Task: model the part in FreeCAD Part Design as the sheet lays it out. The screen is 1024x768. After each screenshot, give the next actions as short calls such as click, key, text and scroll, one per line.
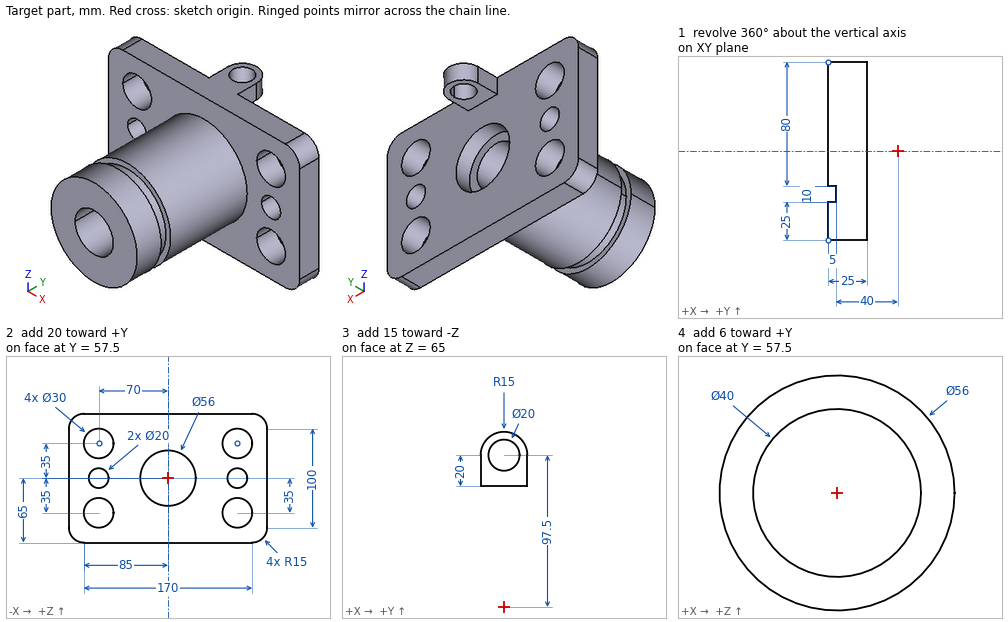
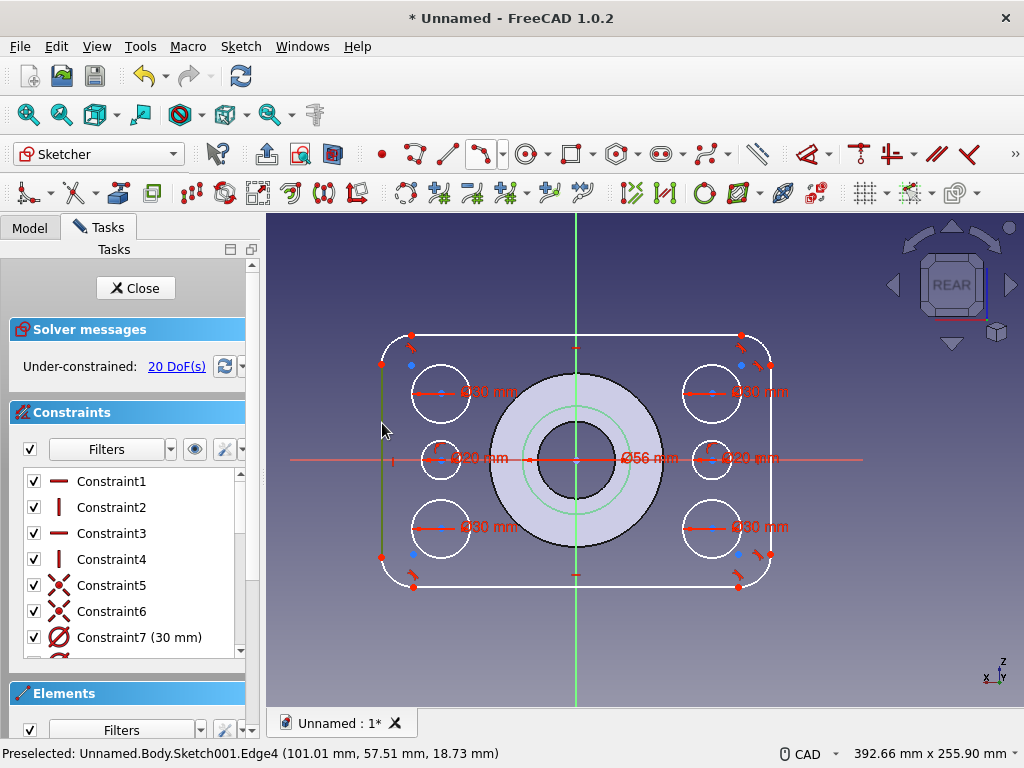
click(398, 339)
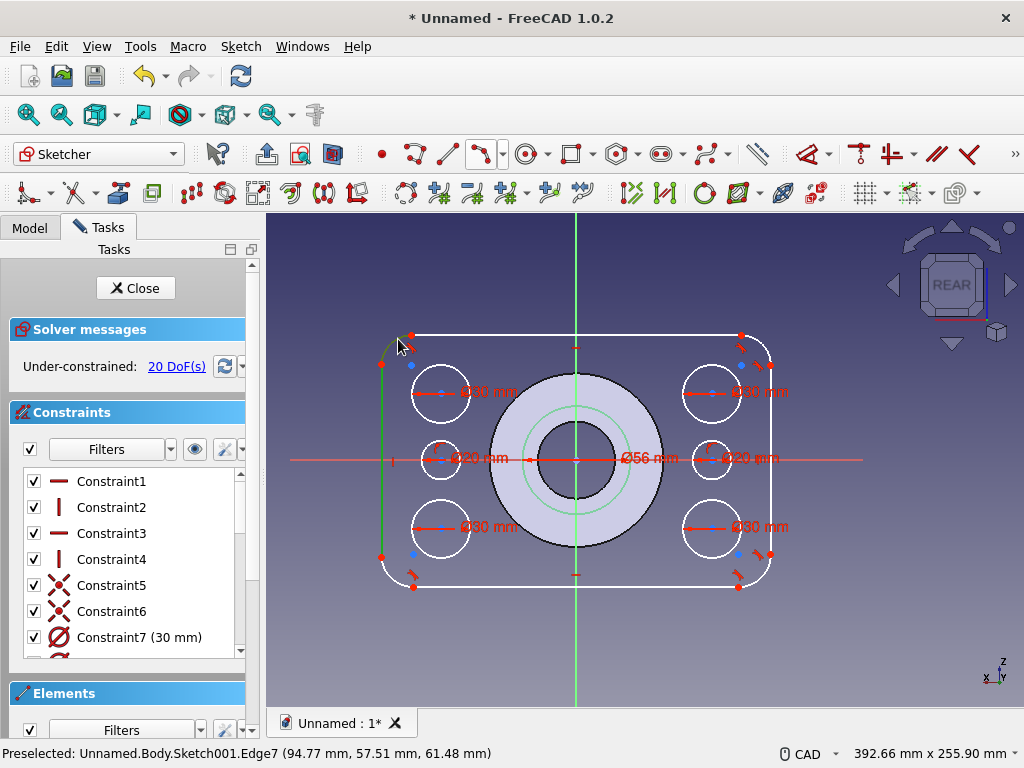
key(t)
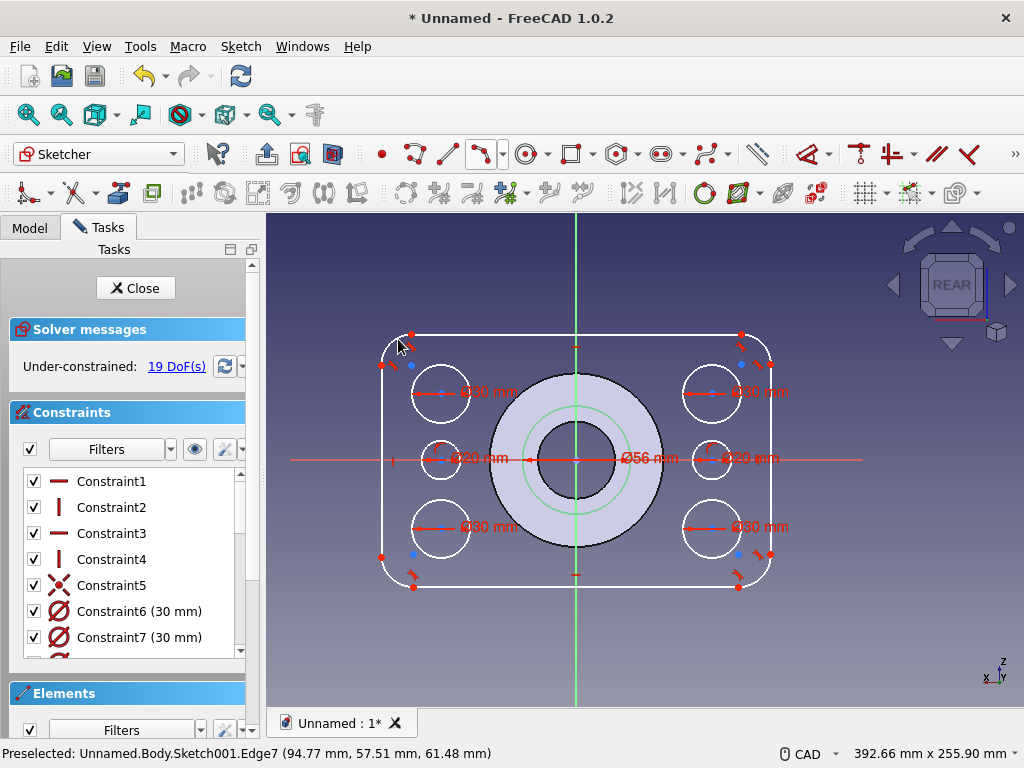
click(382, 423)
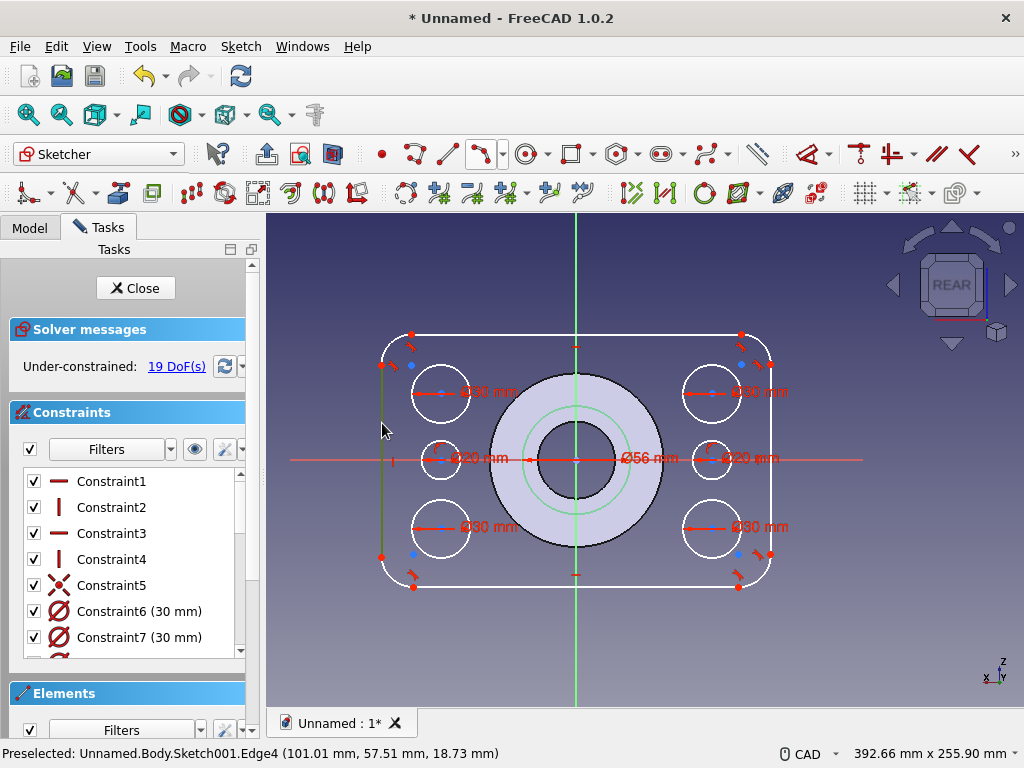
click(386, 571)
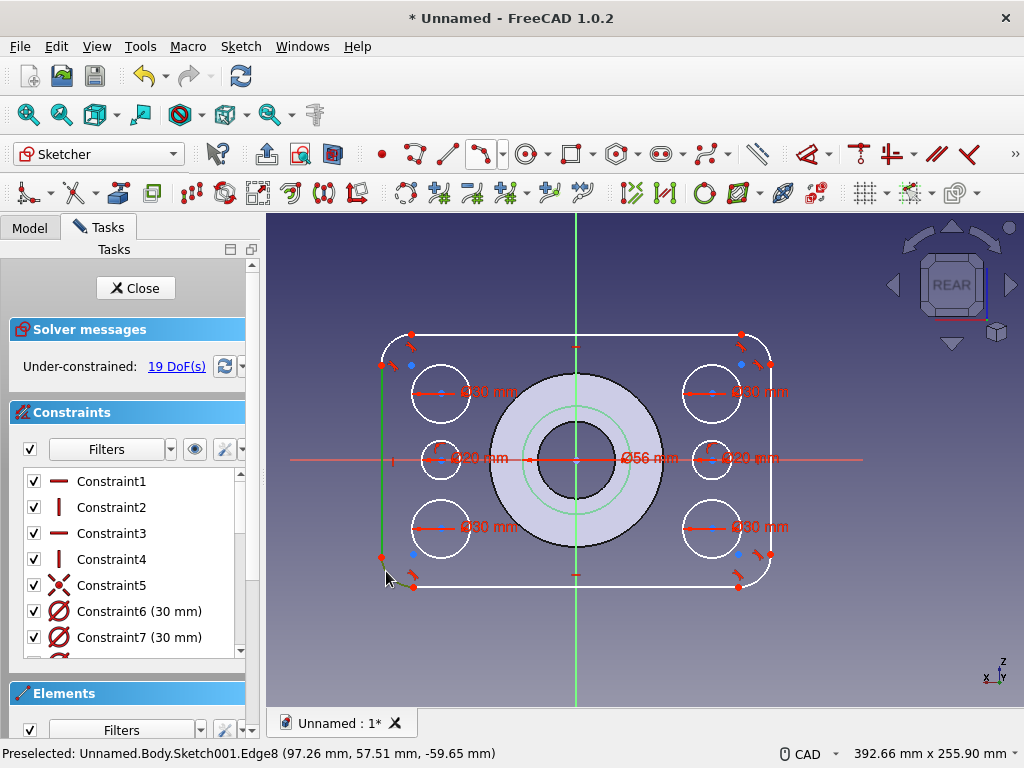
key(t)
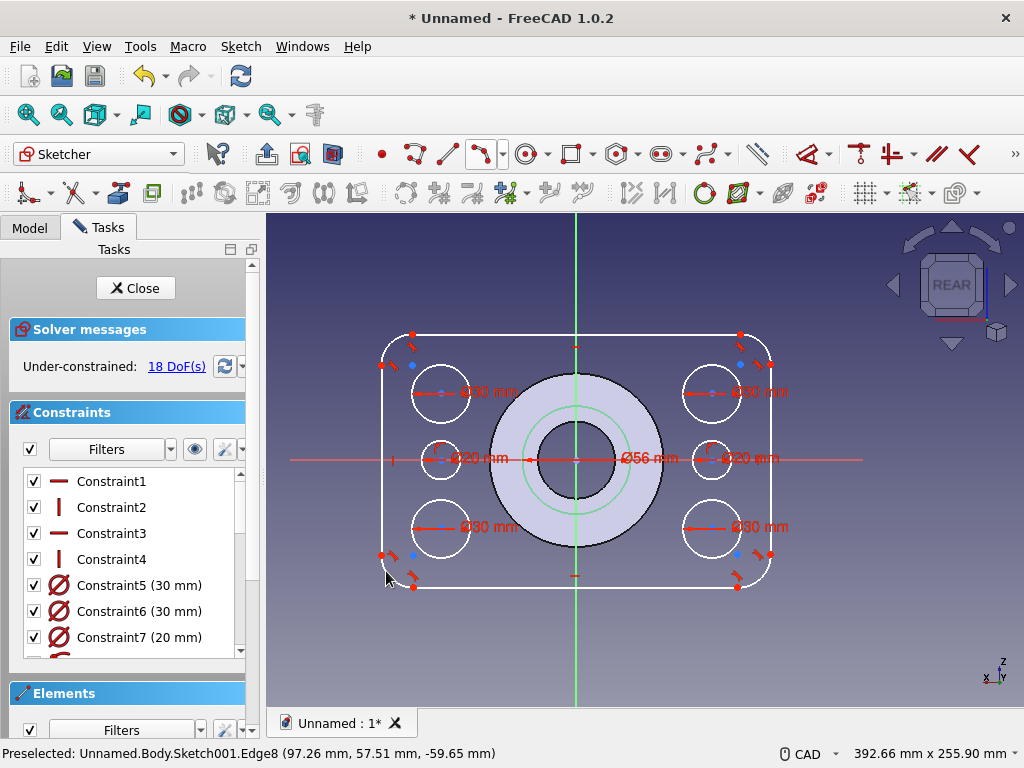
click(753, 584)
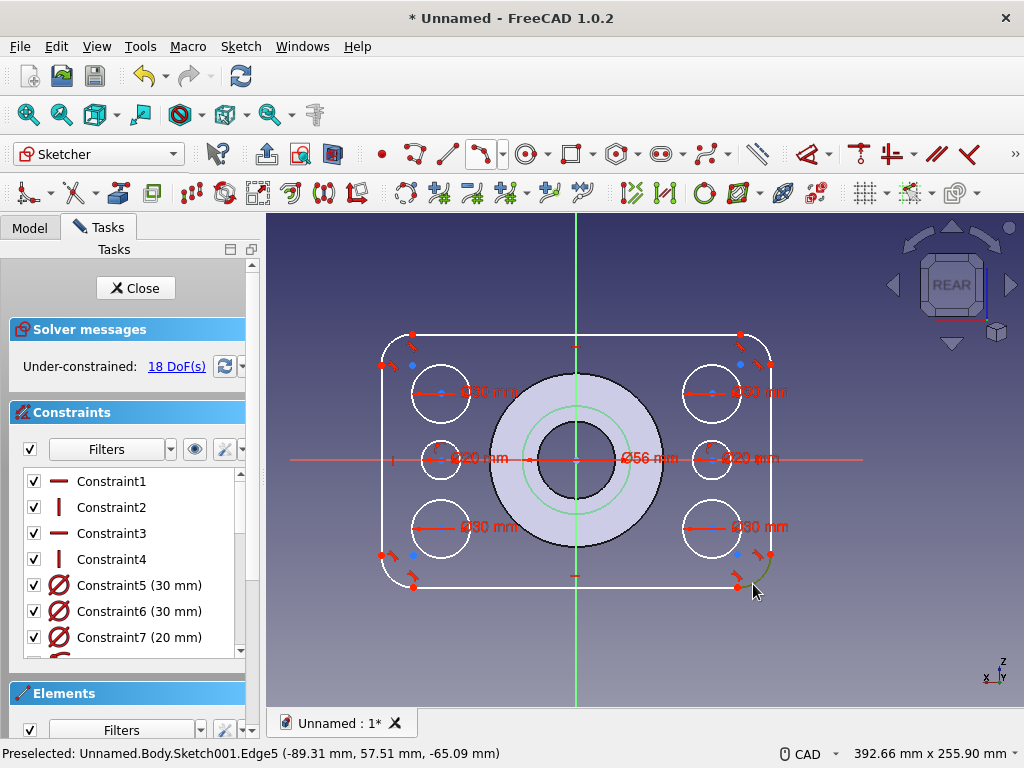
click(768, 351)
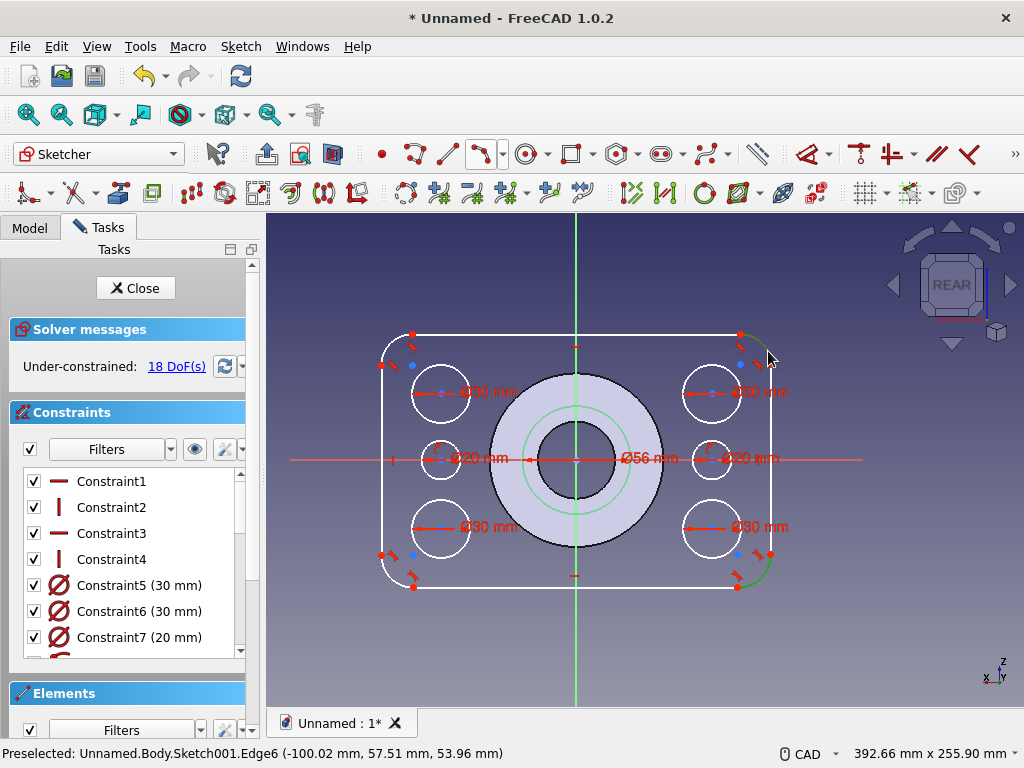
click(398, 338)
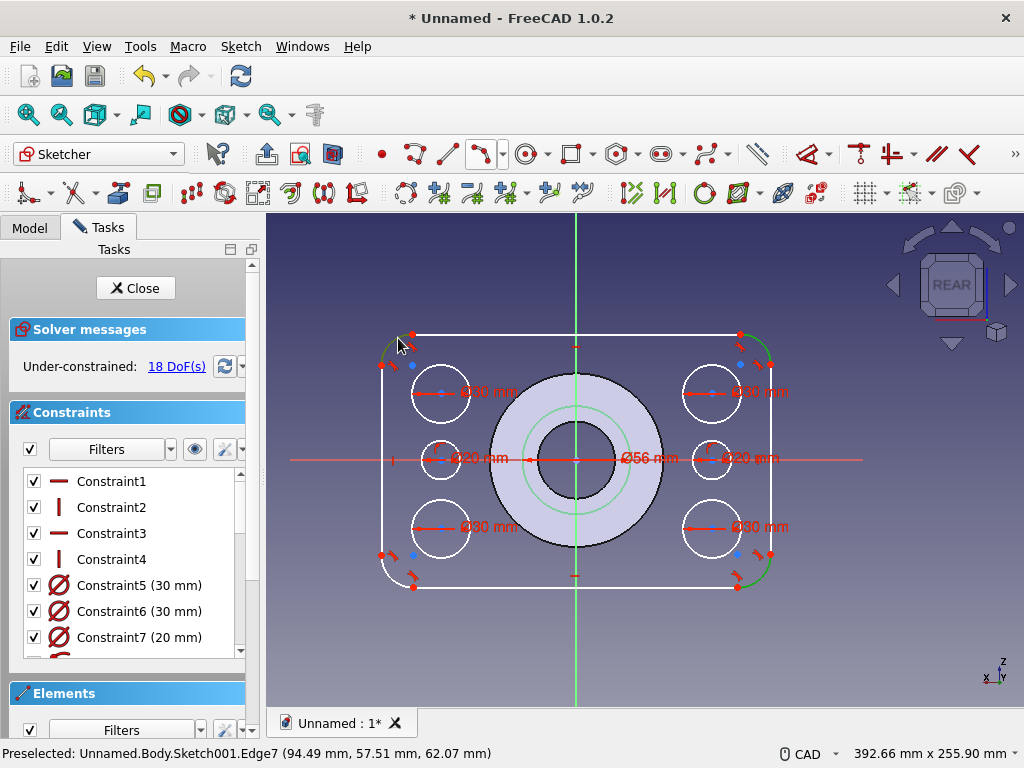
click(385, 570)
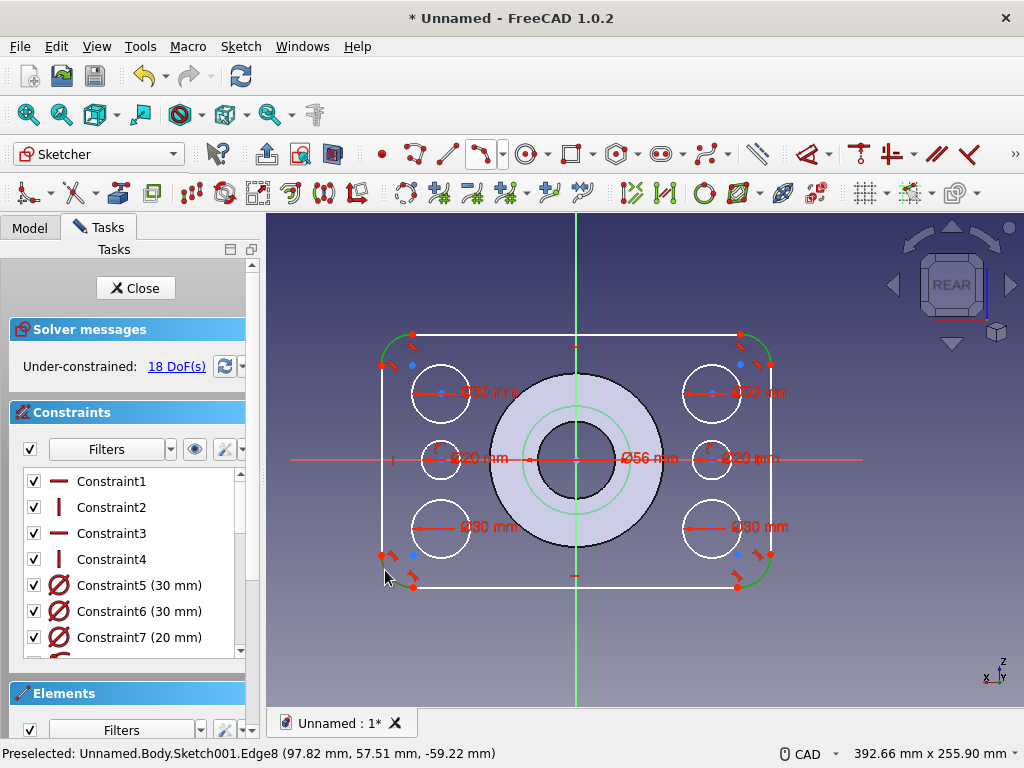
key(e)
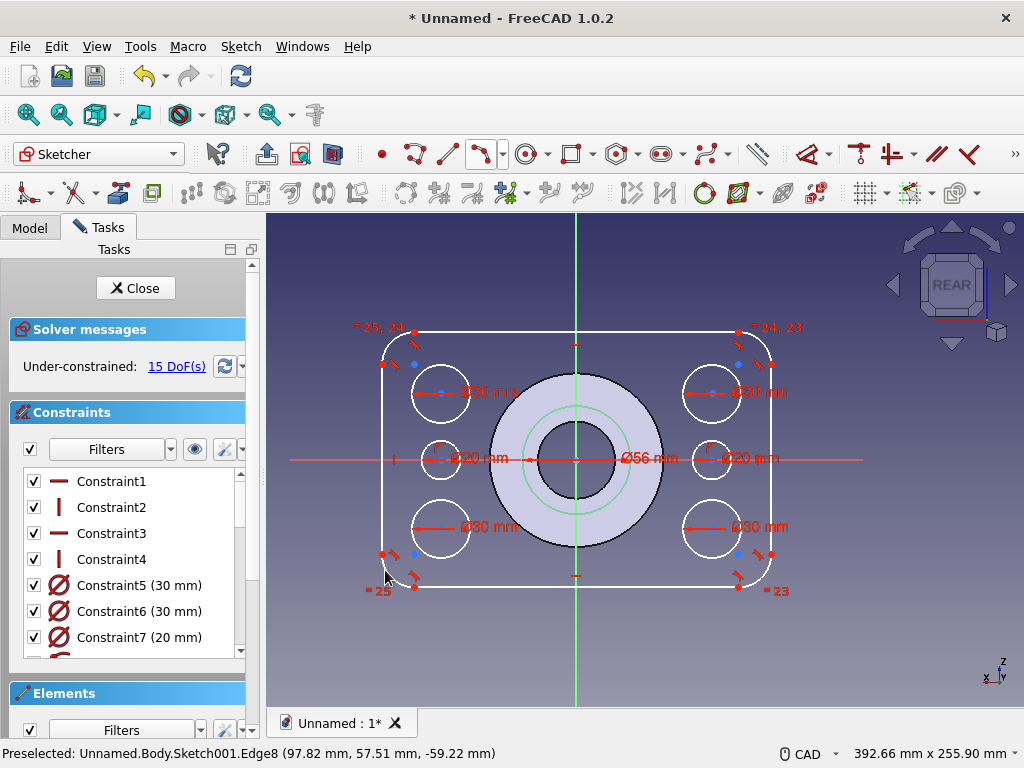
click(441, 394)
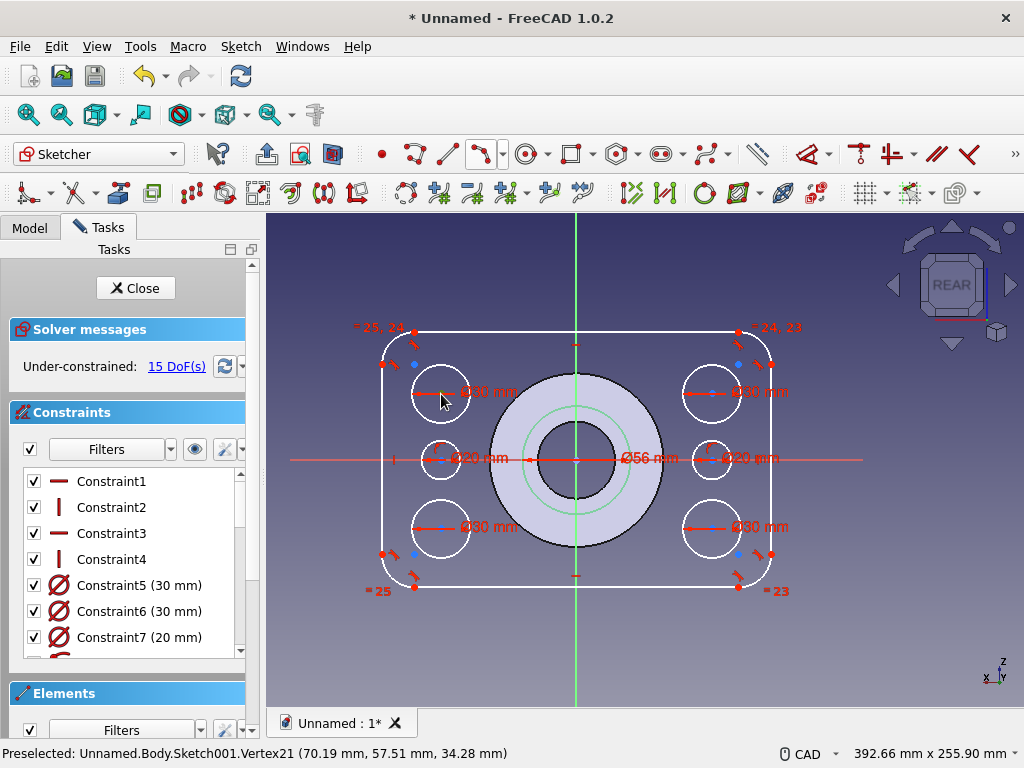
click(441, 460)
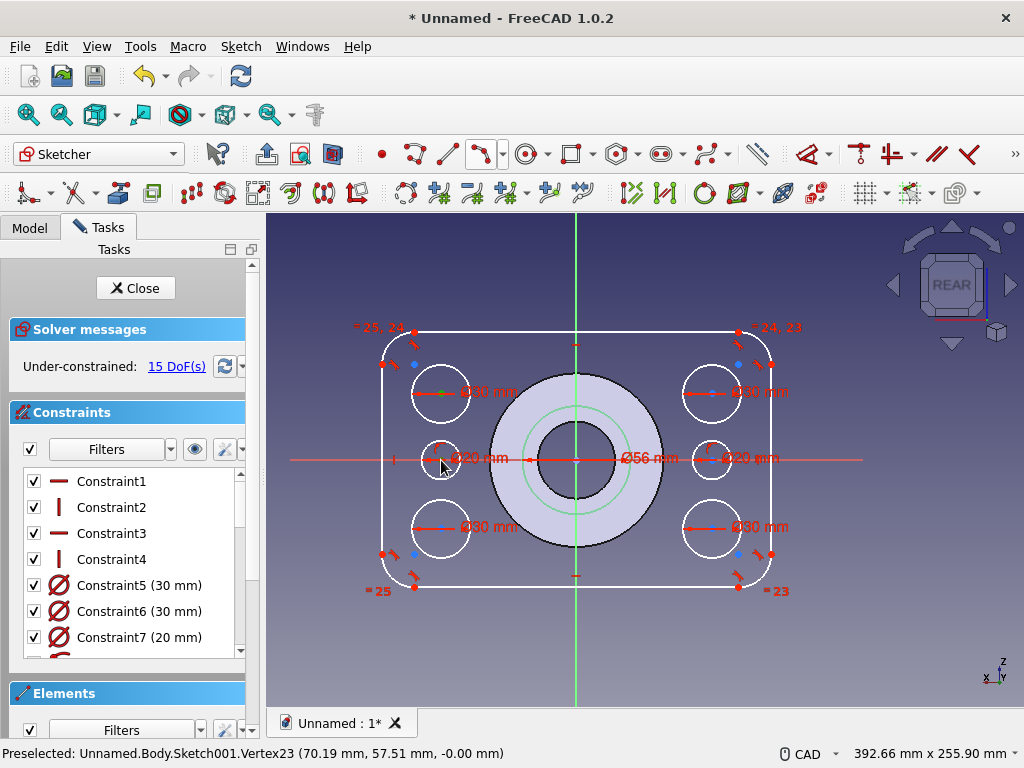
click(914, 154)